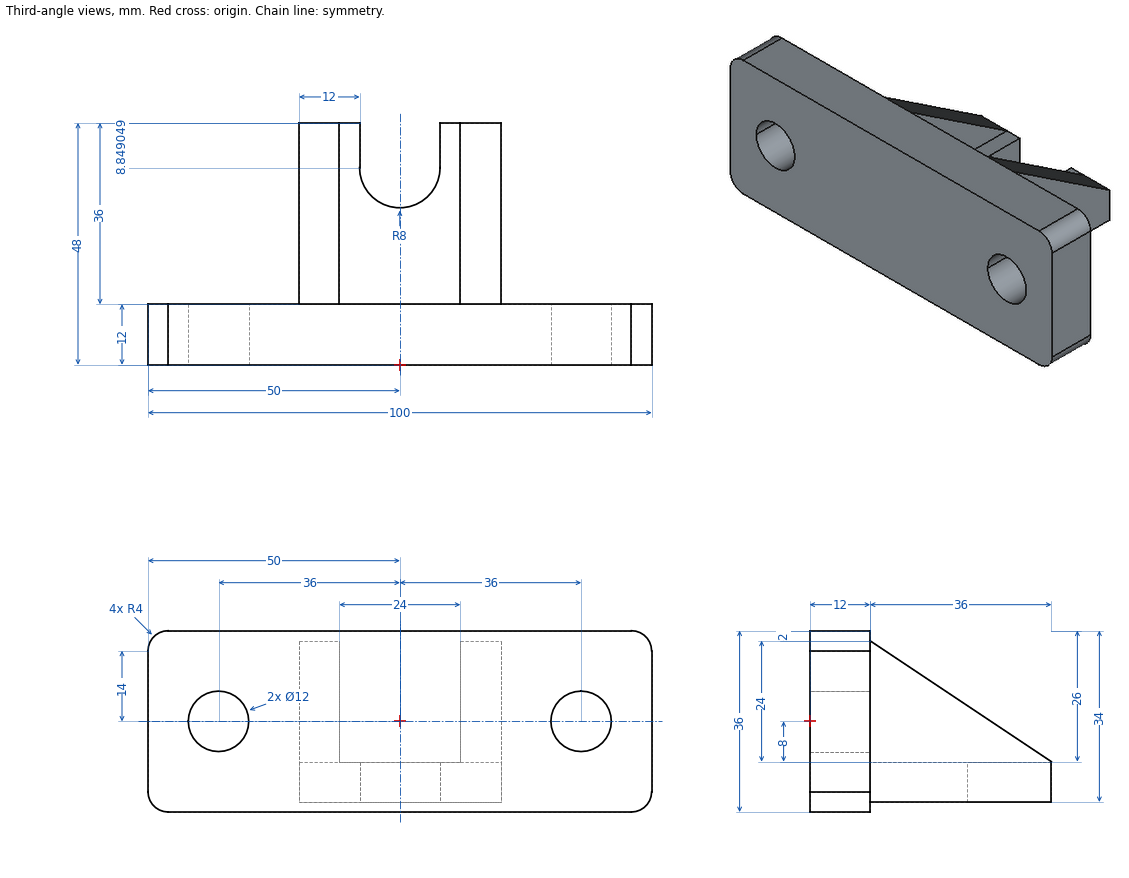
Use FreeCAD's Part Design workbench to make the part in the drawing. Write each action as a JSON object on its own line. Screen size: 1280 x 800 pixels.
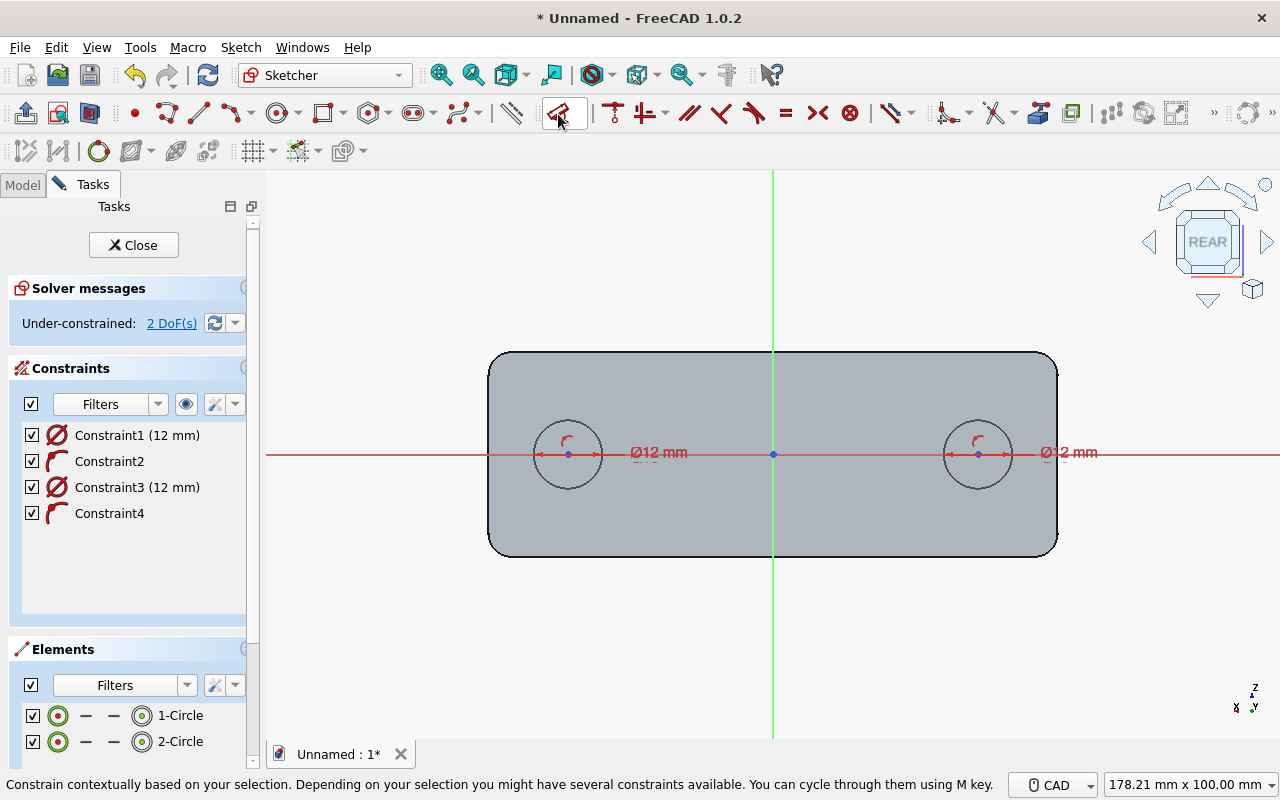
{"action": "left_click", "coordinate": [978, 455]}
{"action": "left_click", "coordinate": [876, 489]}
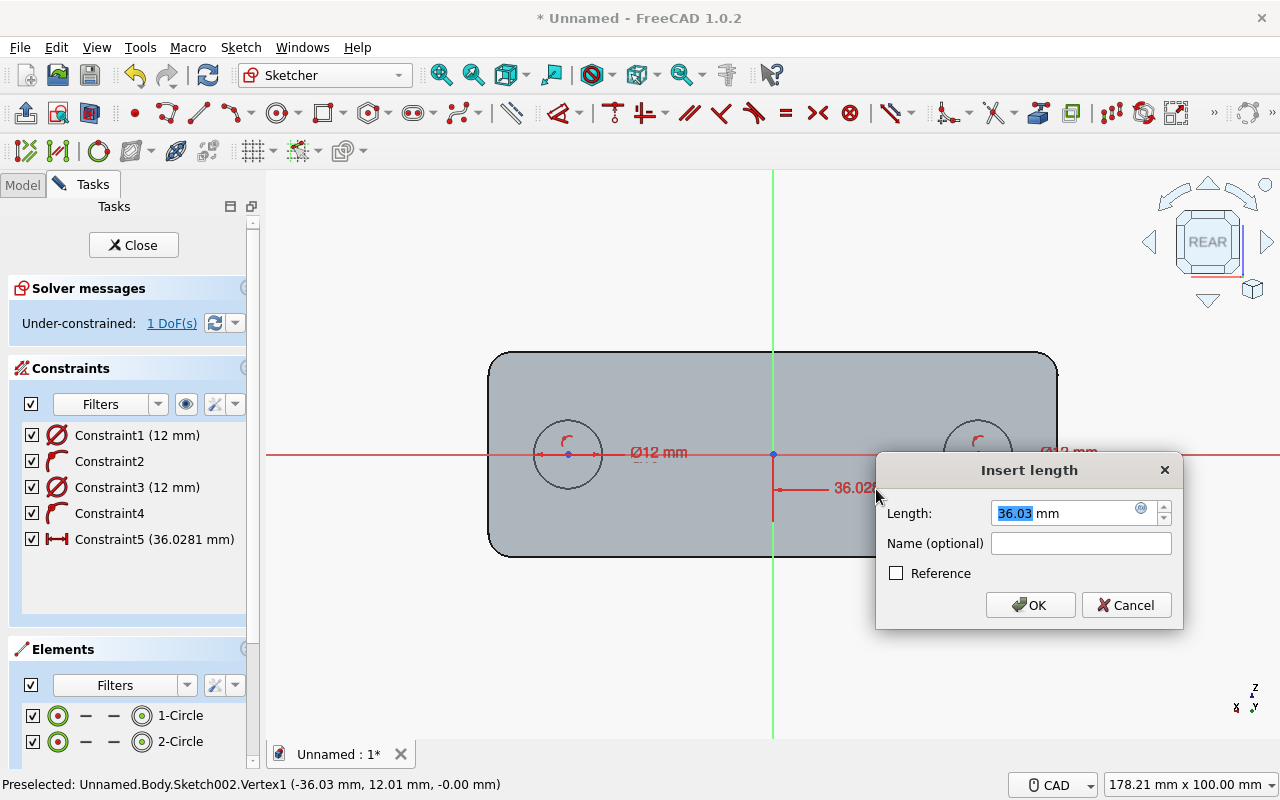
{"action": "type", "text": "36"}
{"action": "key", "text": "Return"}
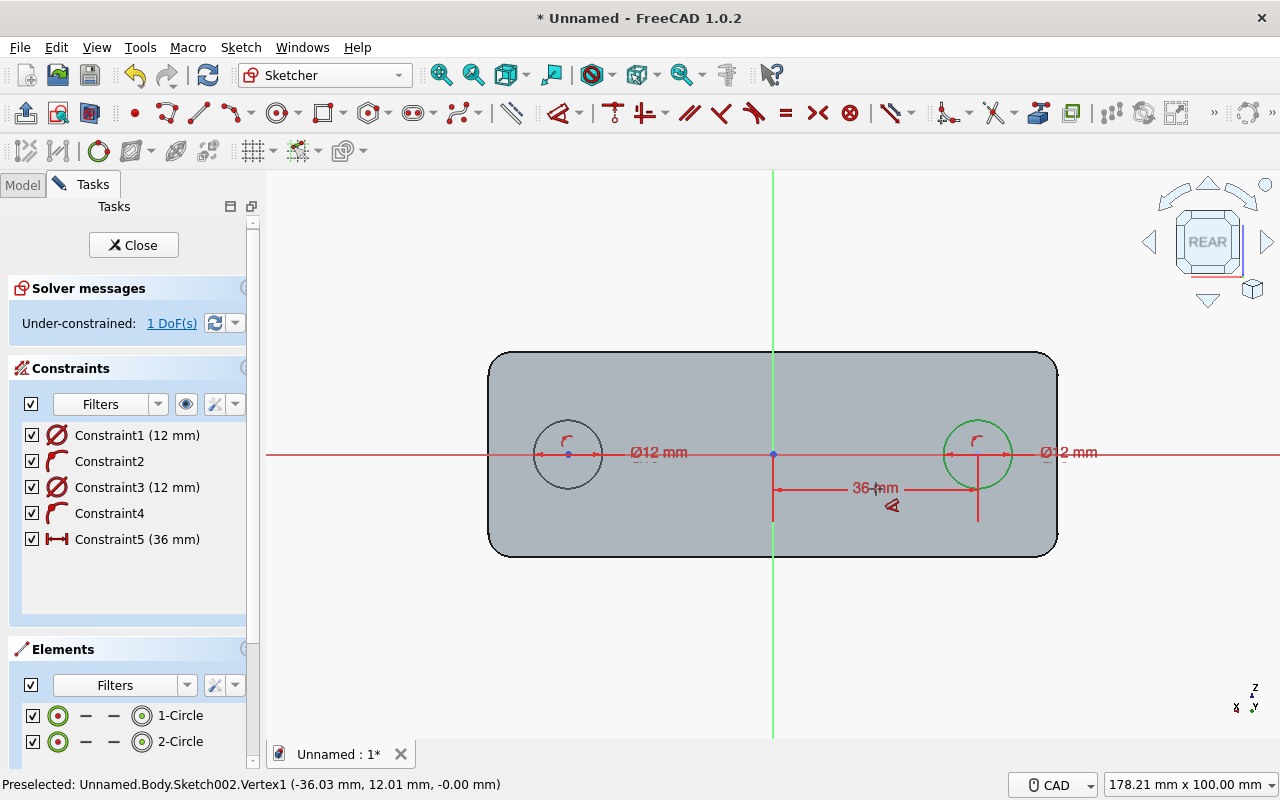
{"action": "left_click", "coordinate": [568, 455]}
{"action": "left_click", "coordinate": [671, 489]}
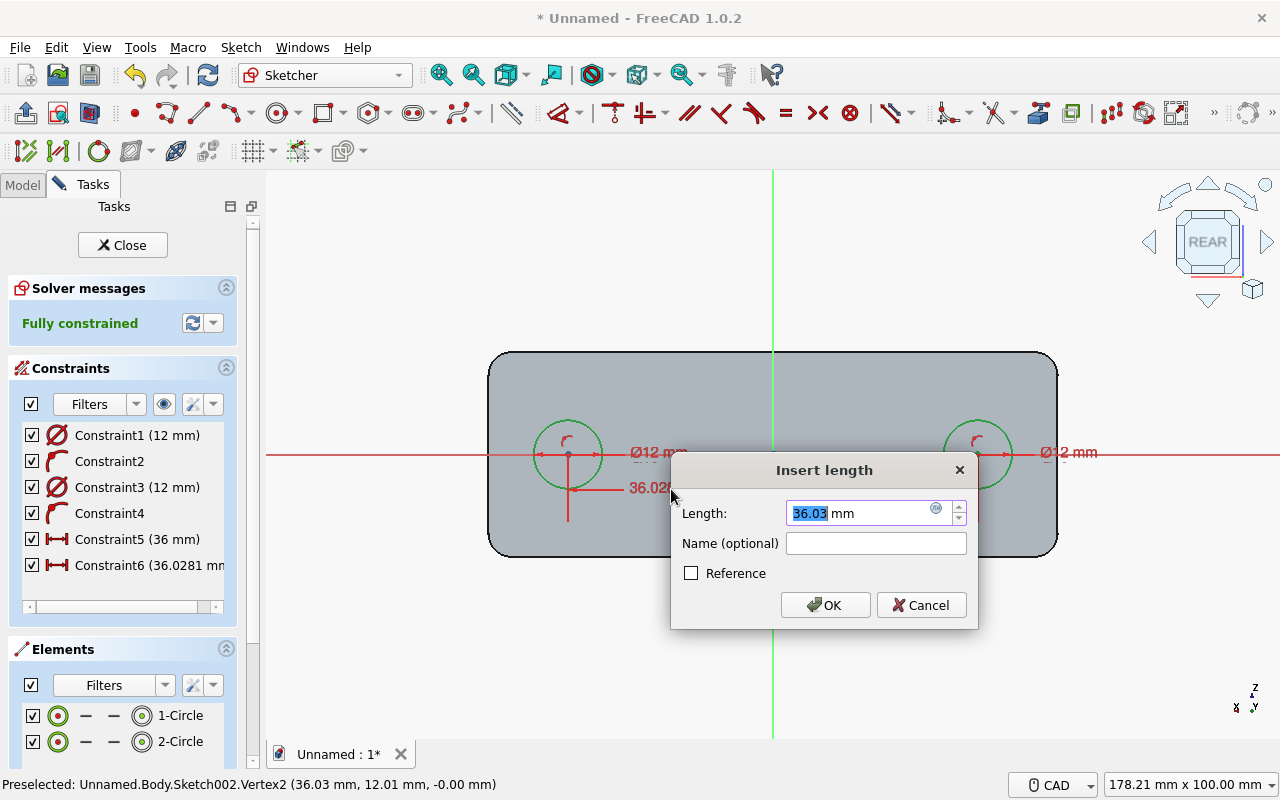
{"action": "type", "text": "36"}
{"action": "key", "text": "Return"}
{"action": "key", "text": "Escape"}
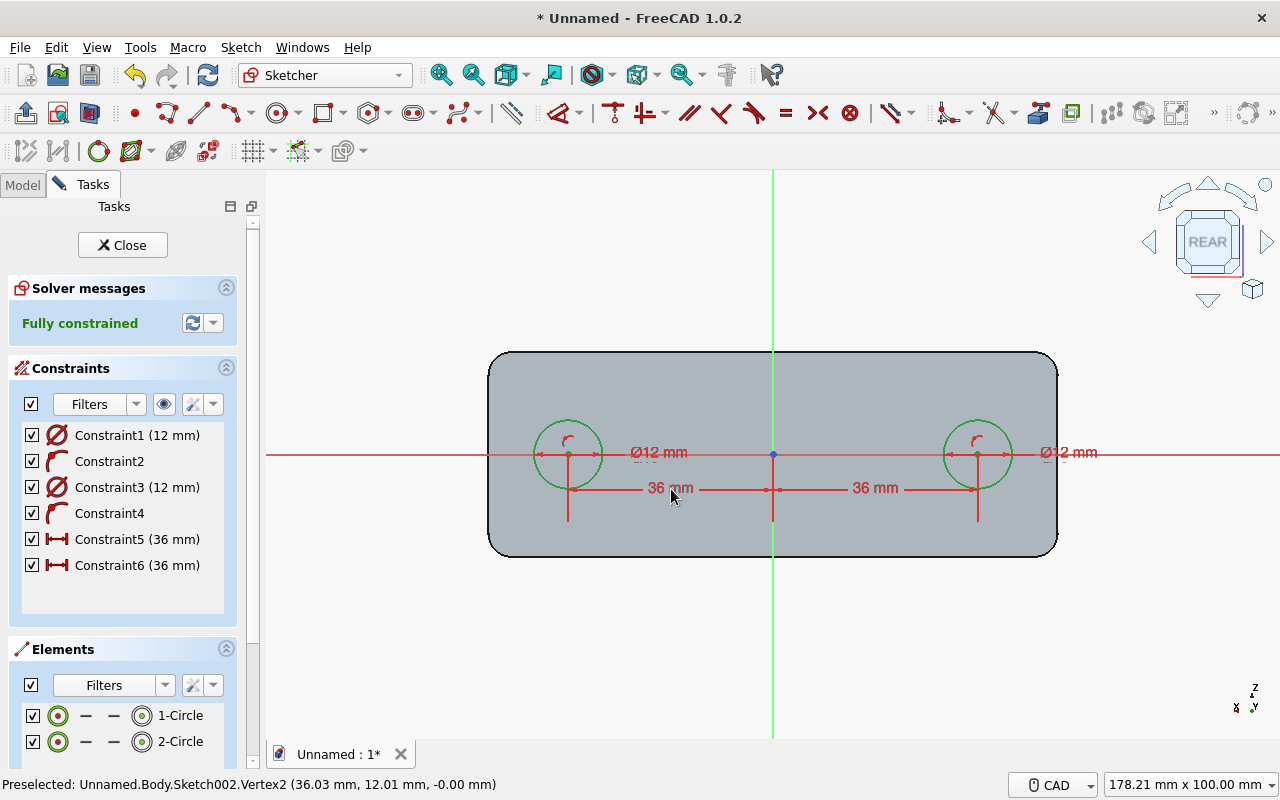
{"action": "left_click", "coordinate": [123, 245]}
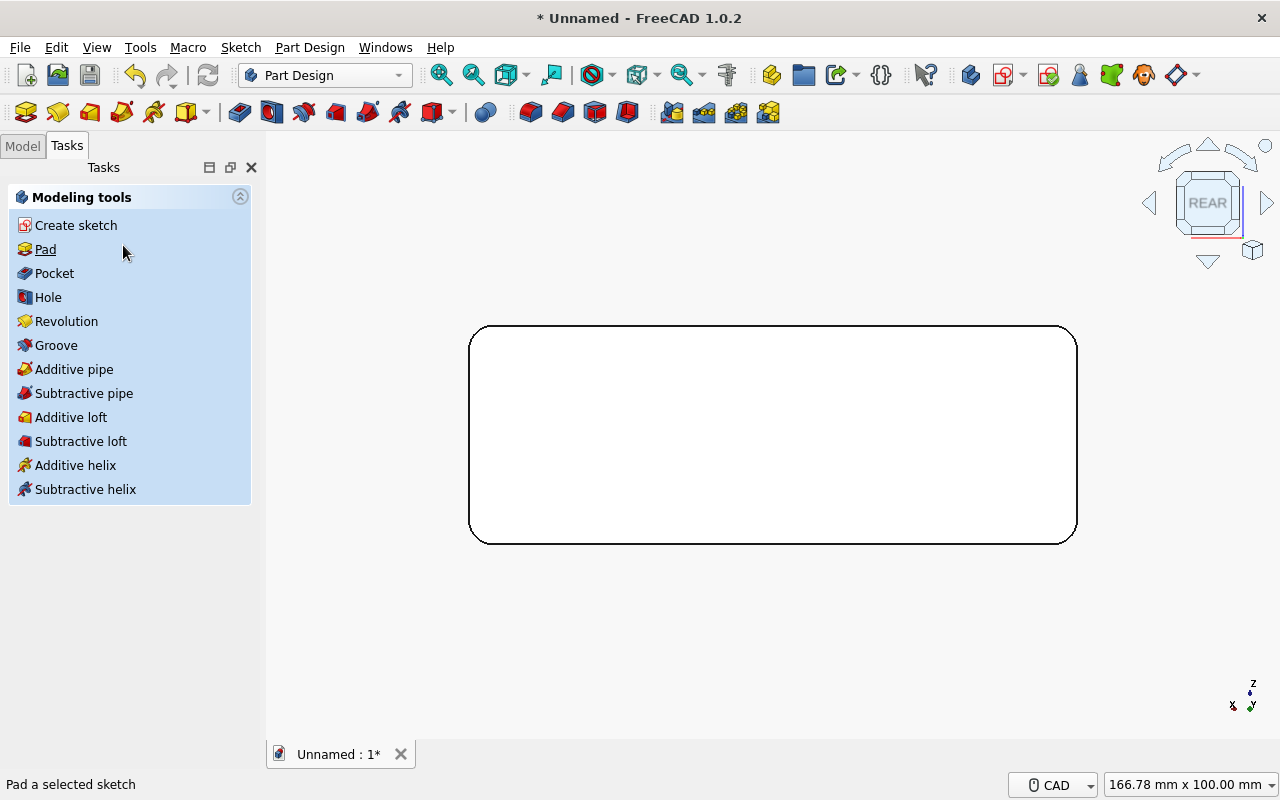
{"action": "left_click", "coordinate": [240, 112]}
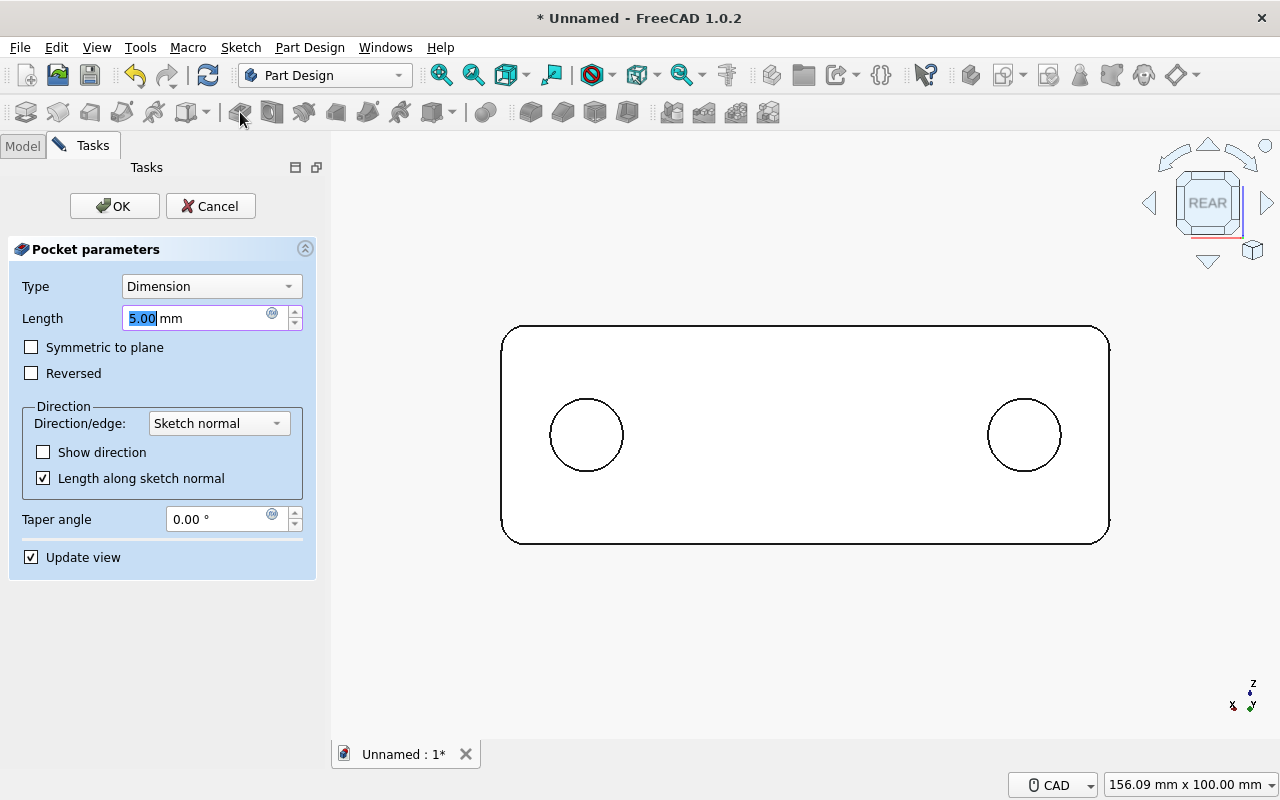
{"action": "type", "text": "36"}
{"action": "key", "text": "Tab"}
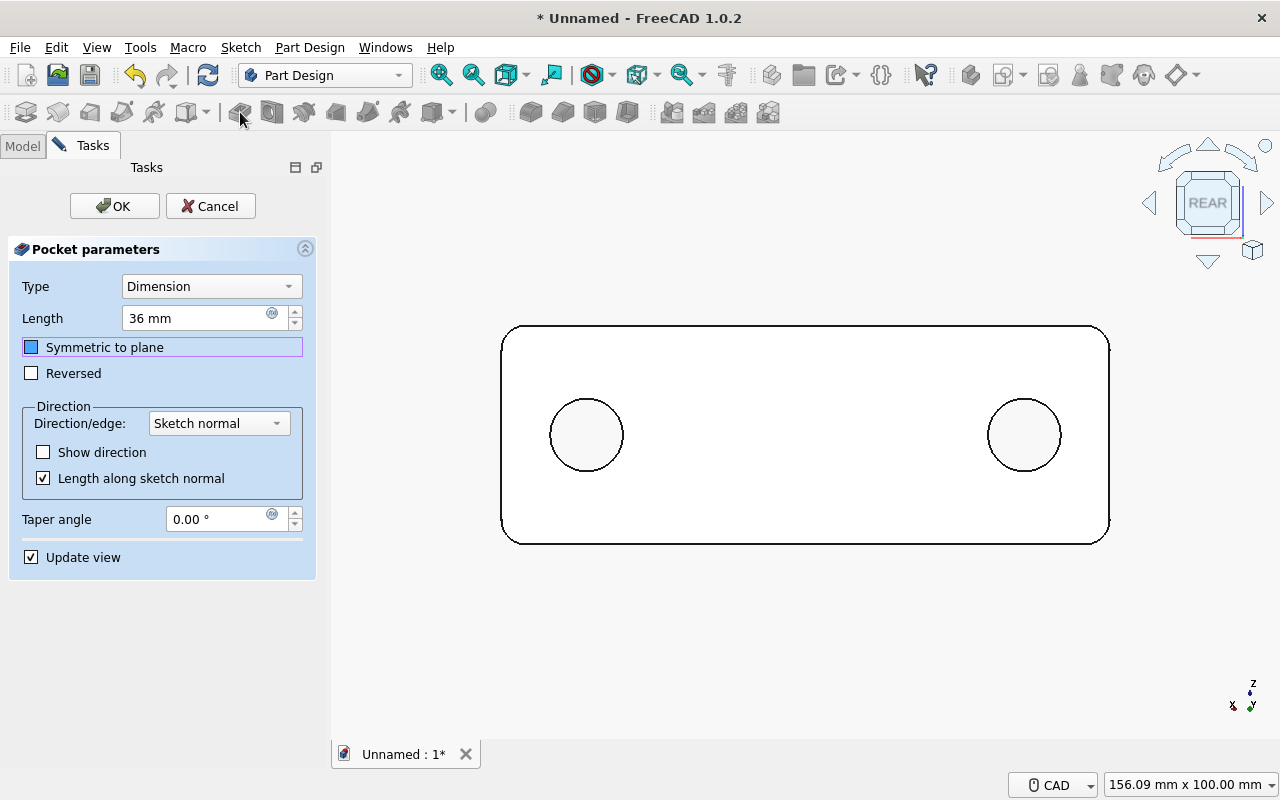
{"action": "left_click", "coordinate": [115, 206]}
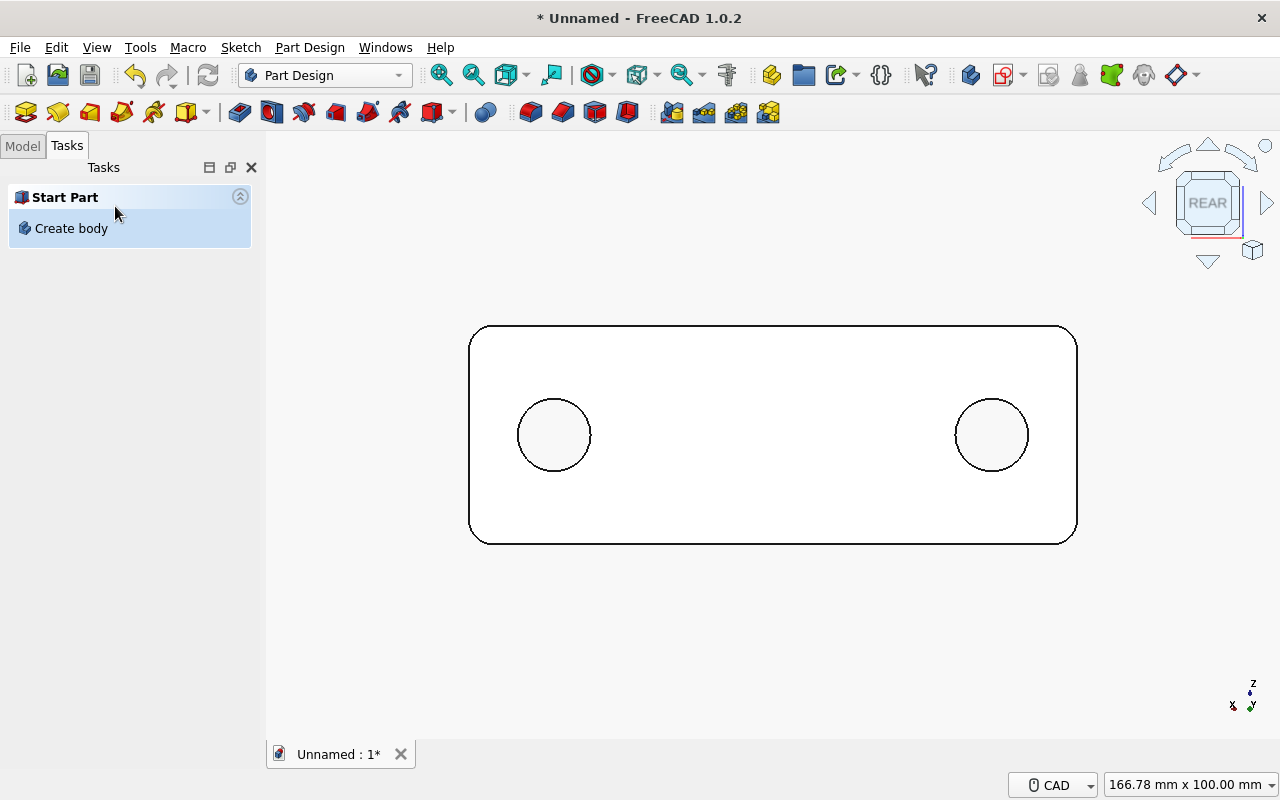
{"action": "key", "text": "0"}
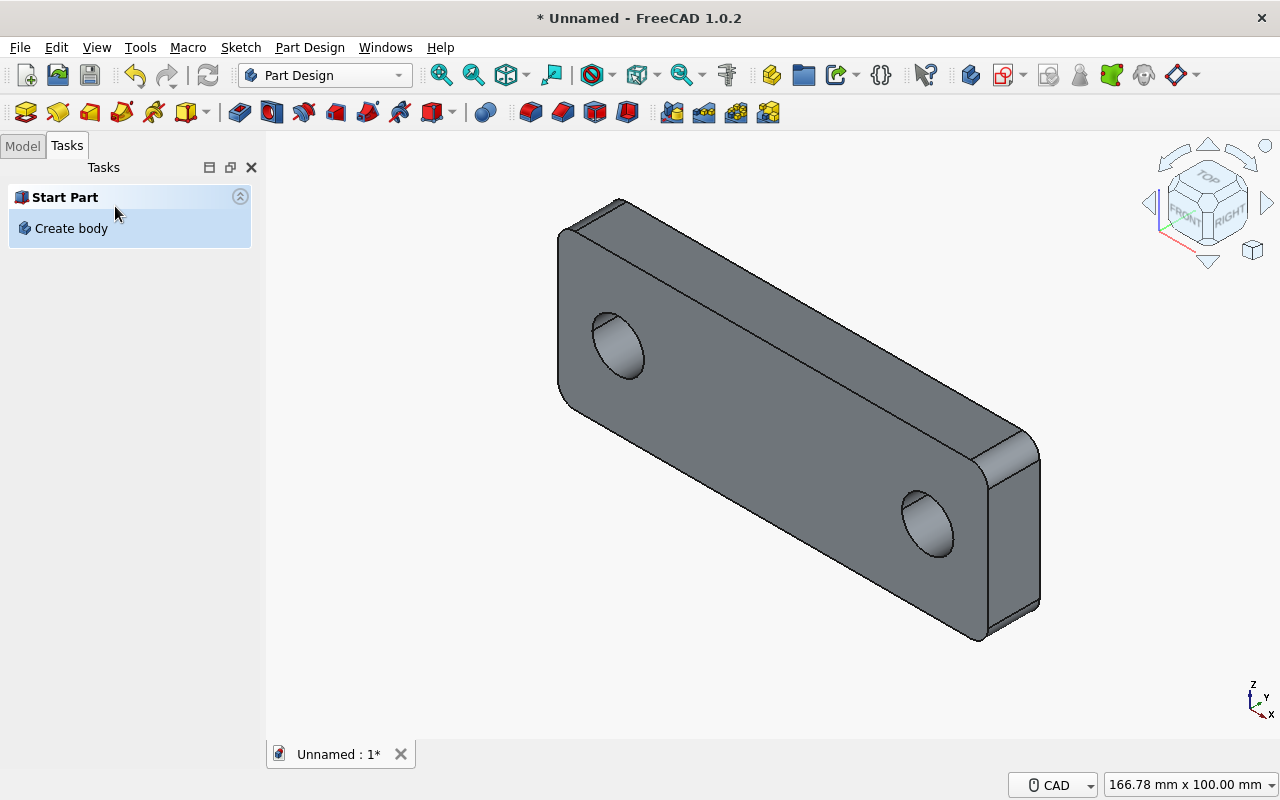
{"action": "left_click", "coordinate": [968, 428]}